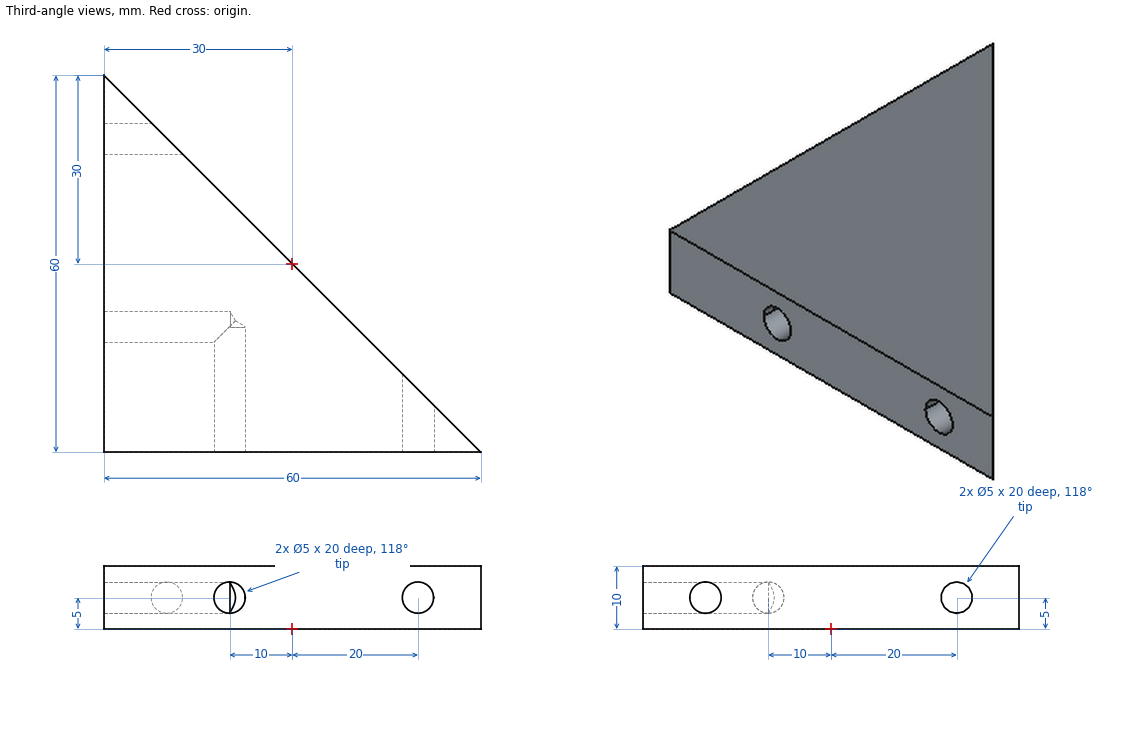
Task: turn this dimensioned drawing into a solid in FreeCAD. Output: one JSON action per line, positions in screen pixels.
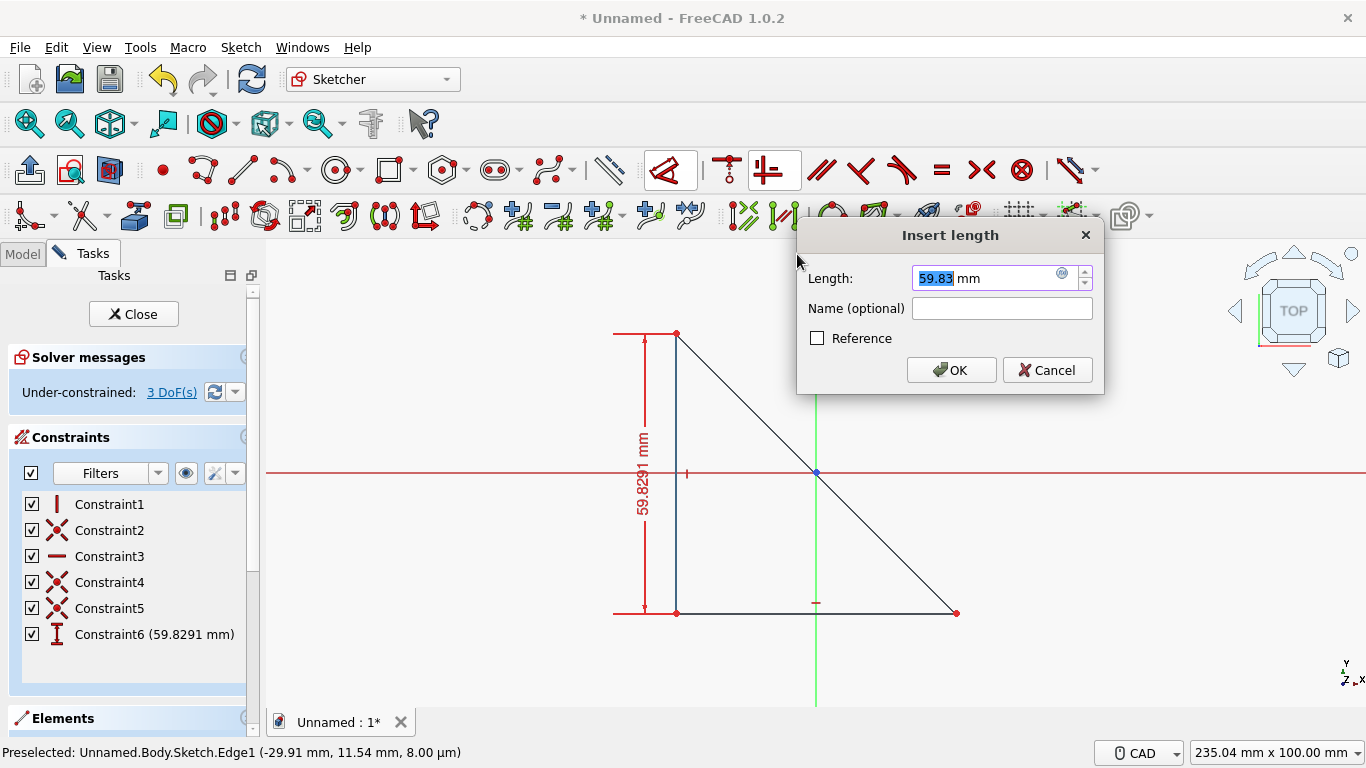
{"action": "type", "text": "60"}
{"action": "key", "text": "Return"}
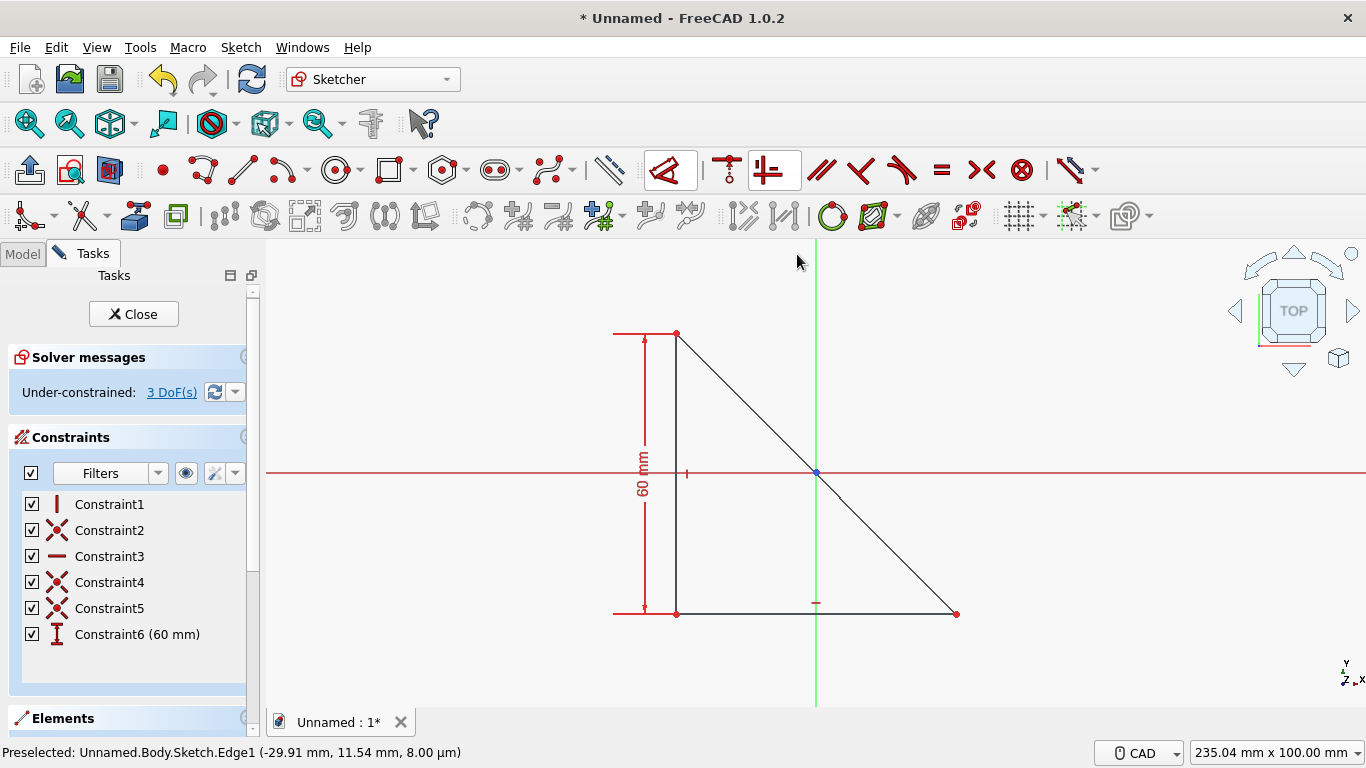
{"action": "left_click", "coordinate": [760, 614]}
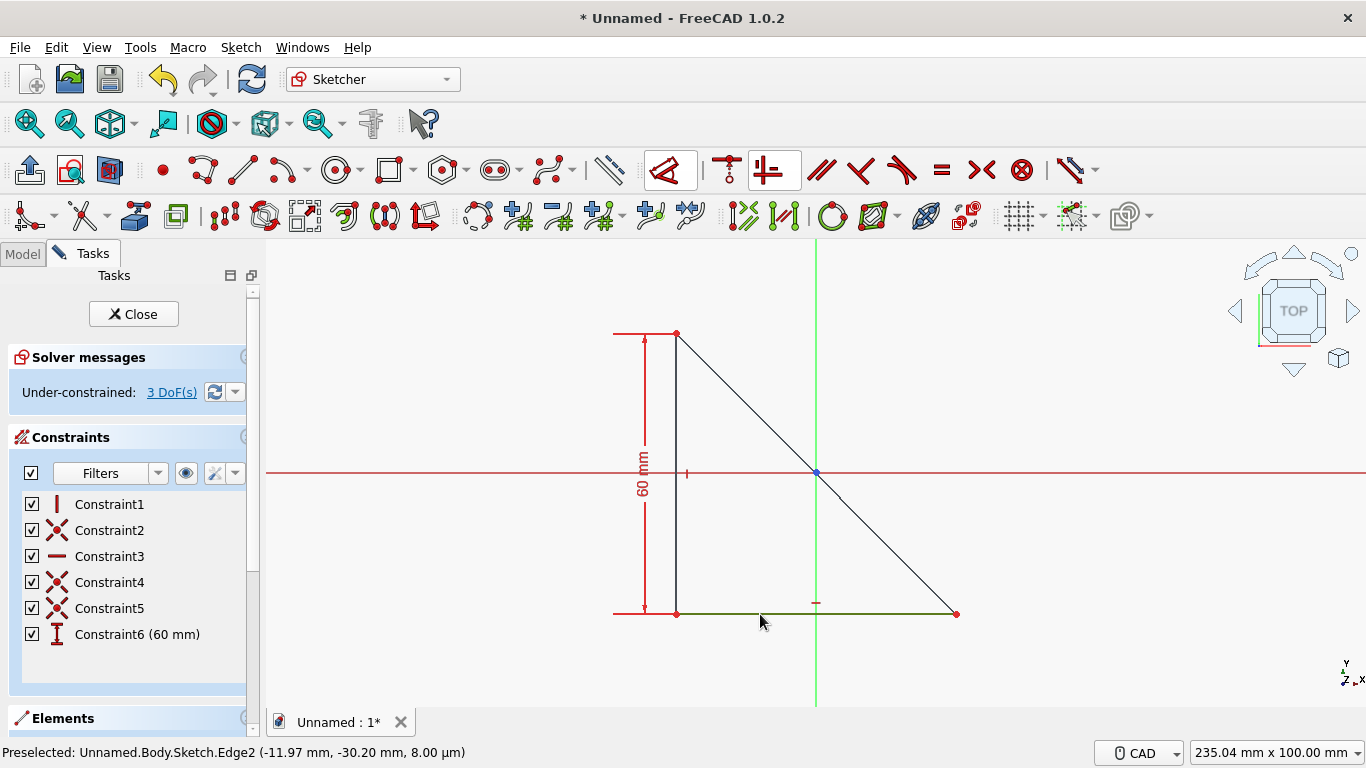
{"action": "key", "text": "l"}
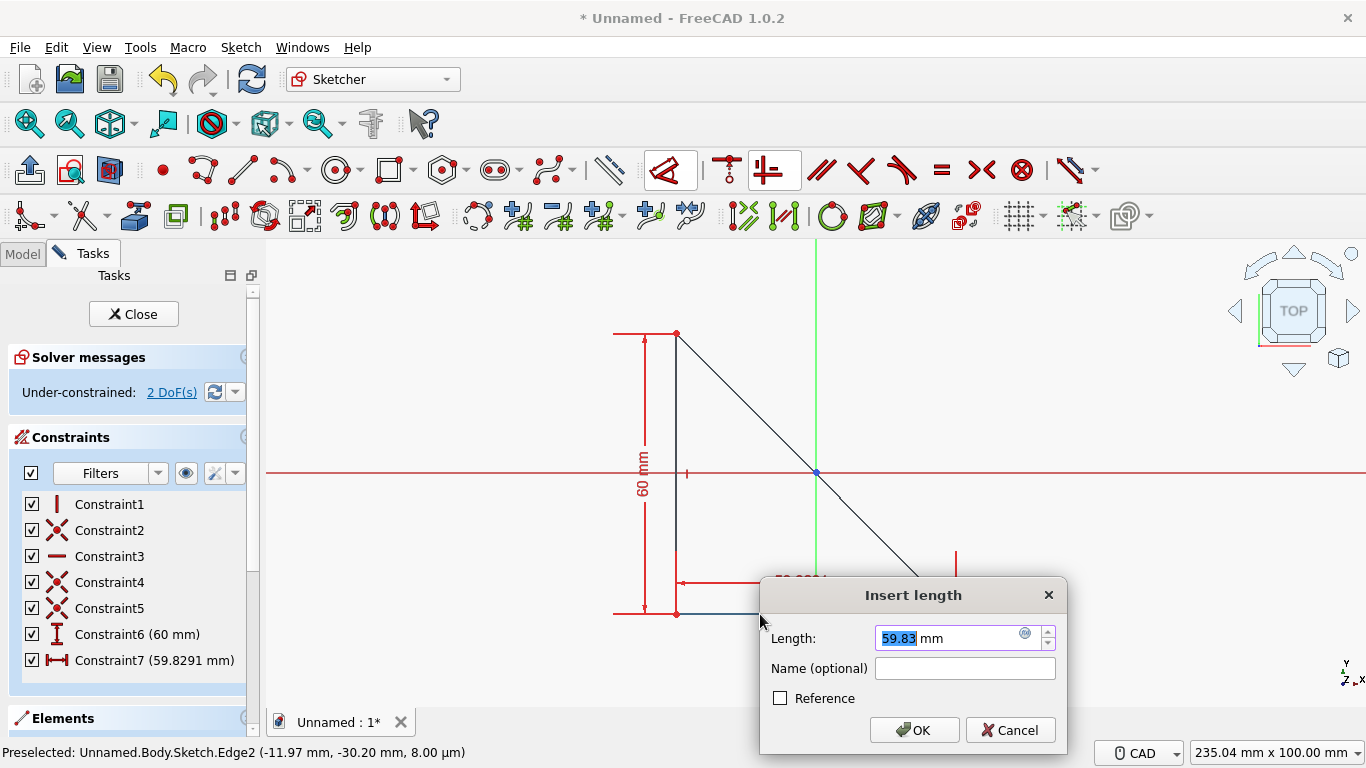
{"action": "type", "text": "60"}
{"action": "key", "text": "Return"}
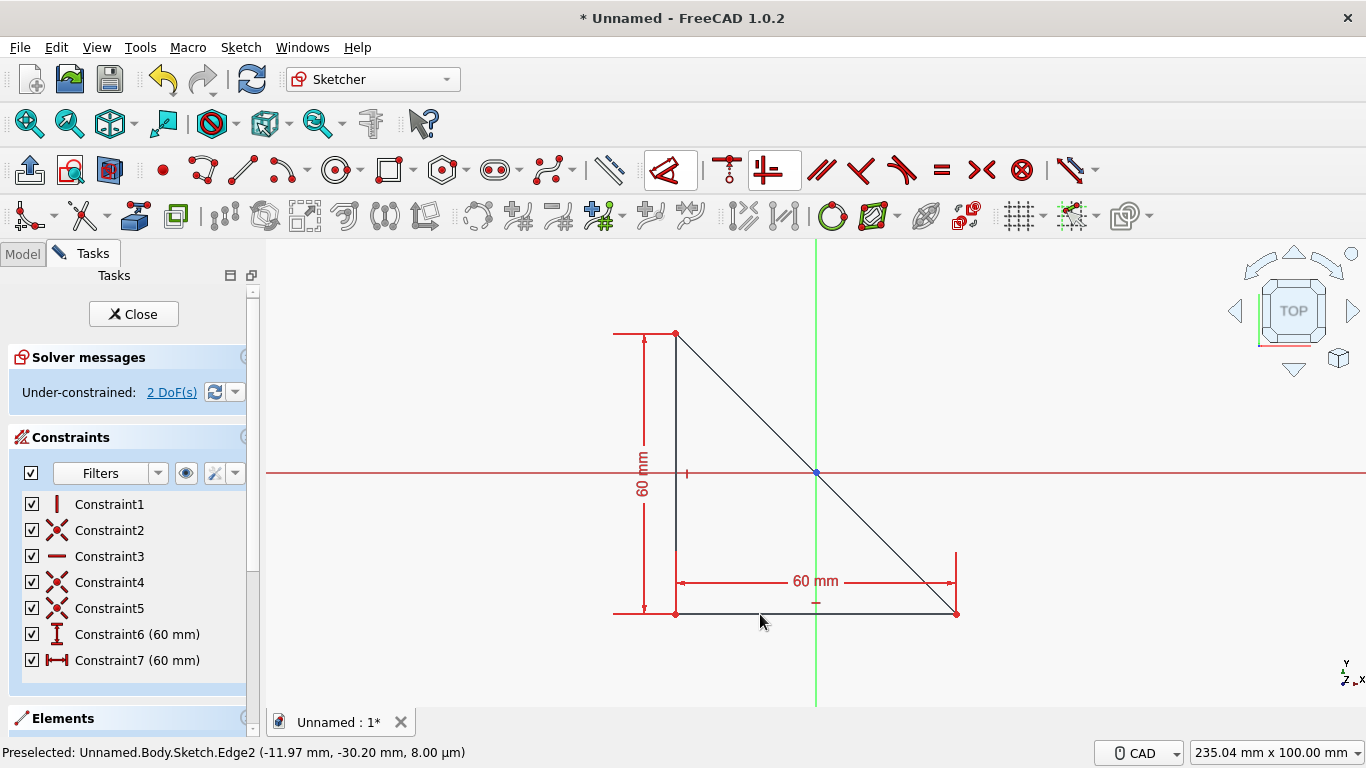
{"action": "left_click", "coordinate": [676, 334]}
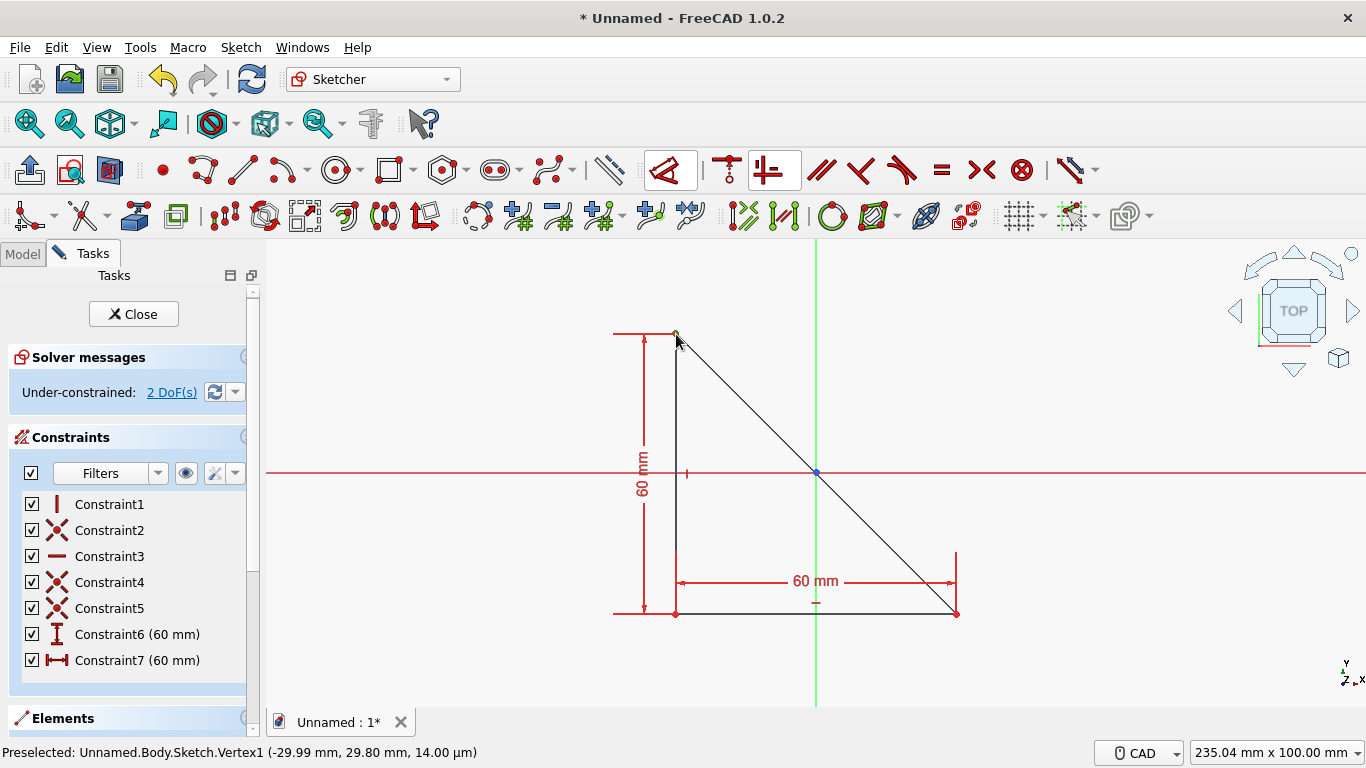
{"action": "key", "text": "l"}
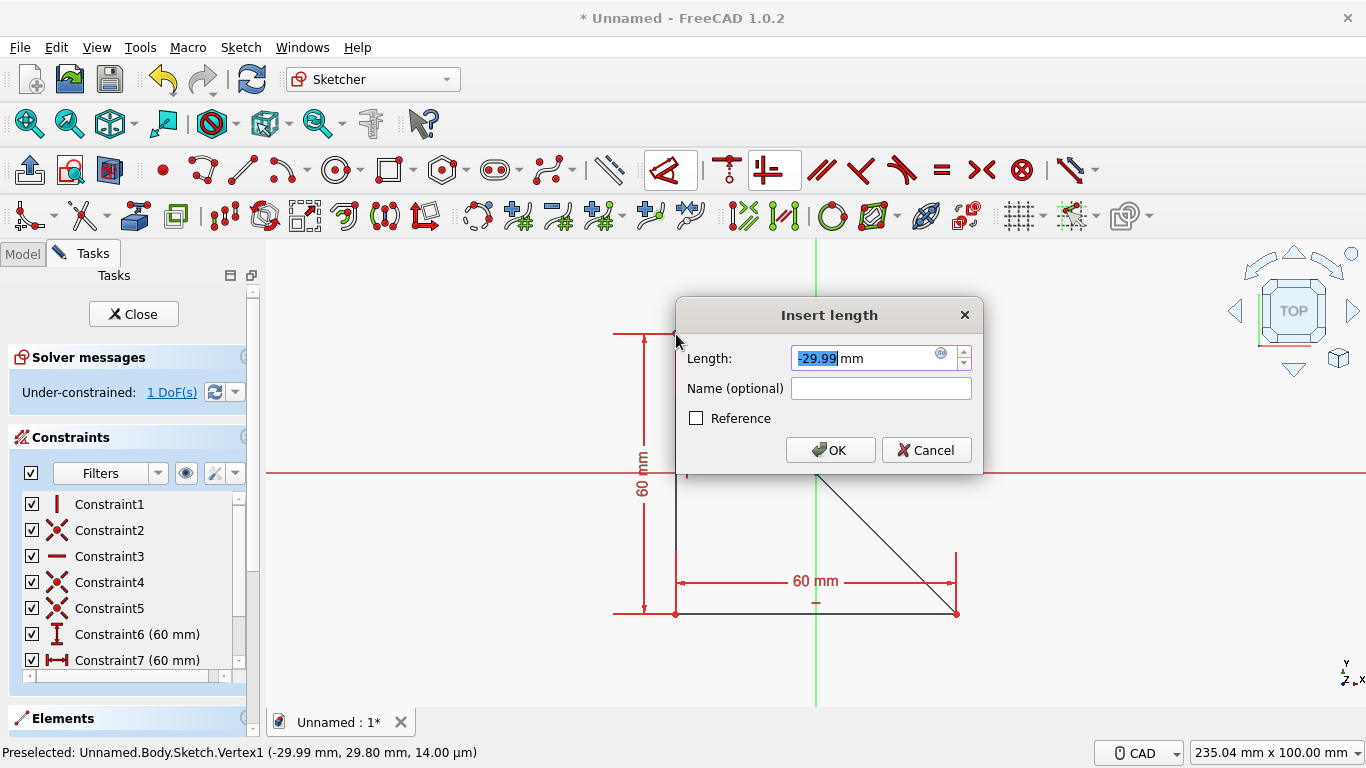
{"action": "type", "text": "-30"}
{"action": "key", "text": "Return"}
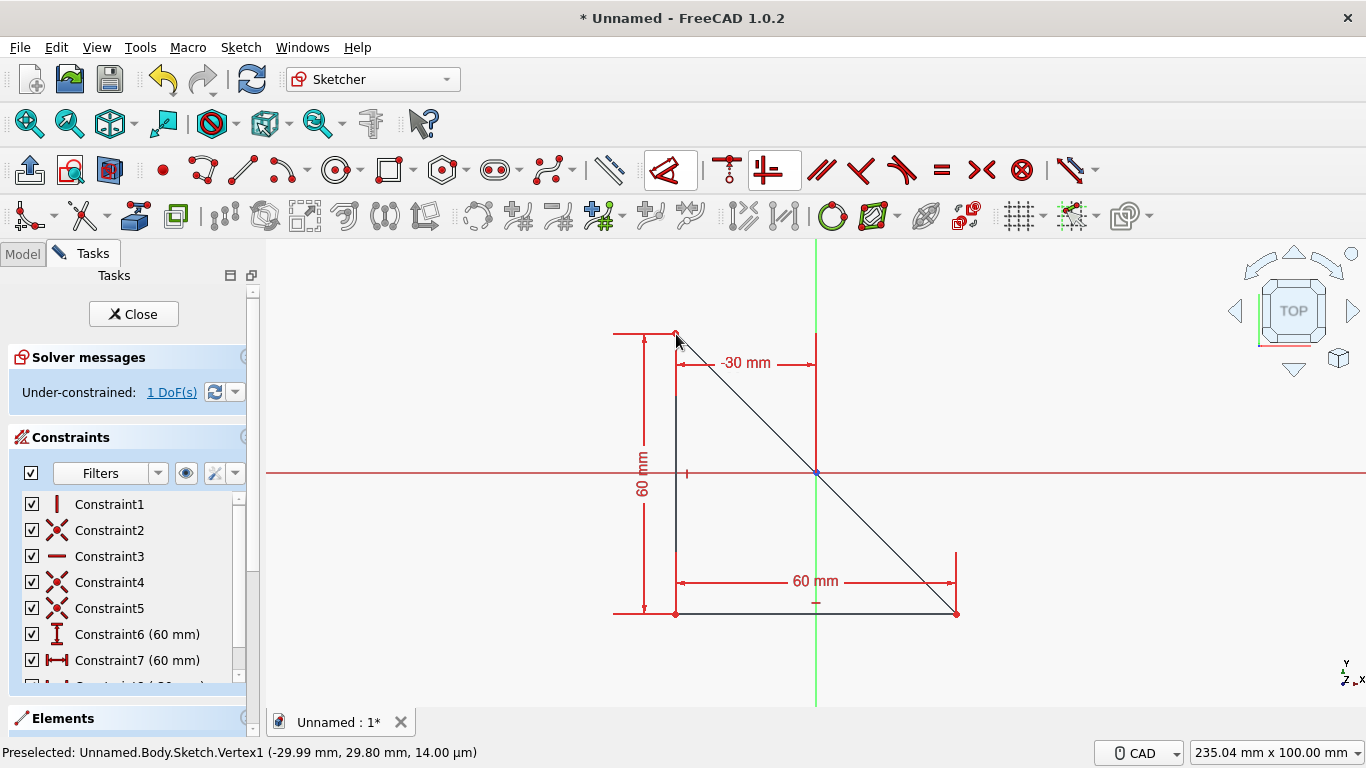
{"action": "left_click", "coordinate": [676, 334]}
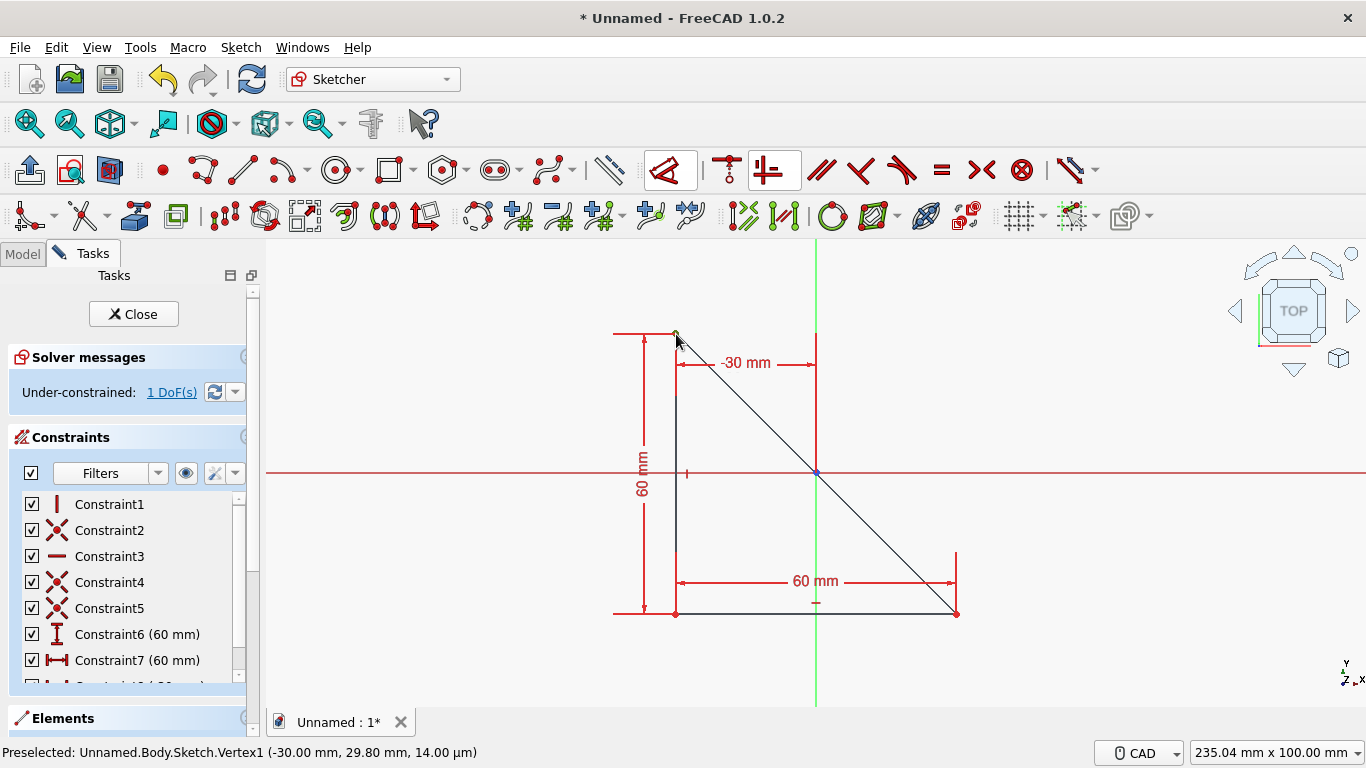
{"action": "key", "text": "i"}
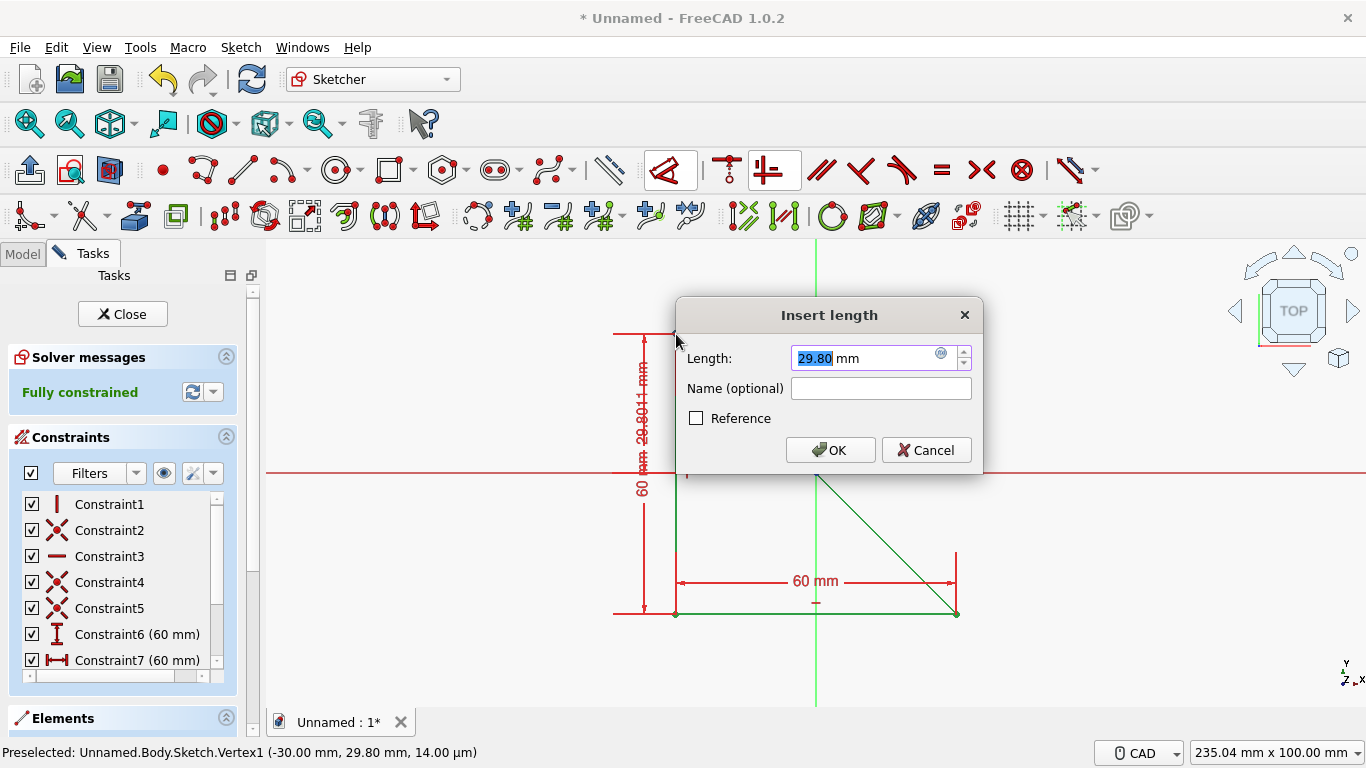
{"action": "type", "text": "30"}
{"action": "key", "text": "Return"}